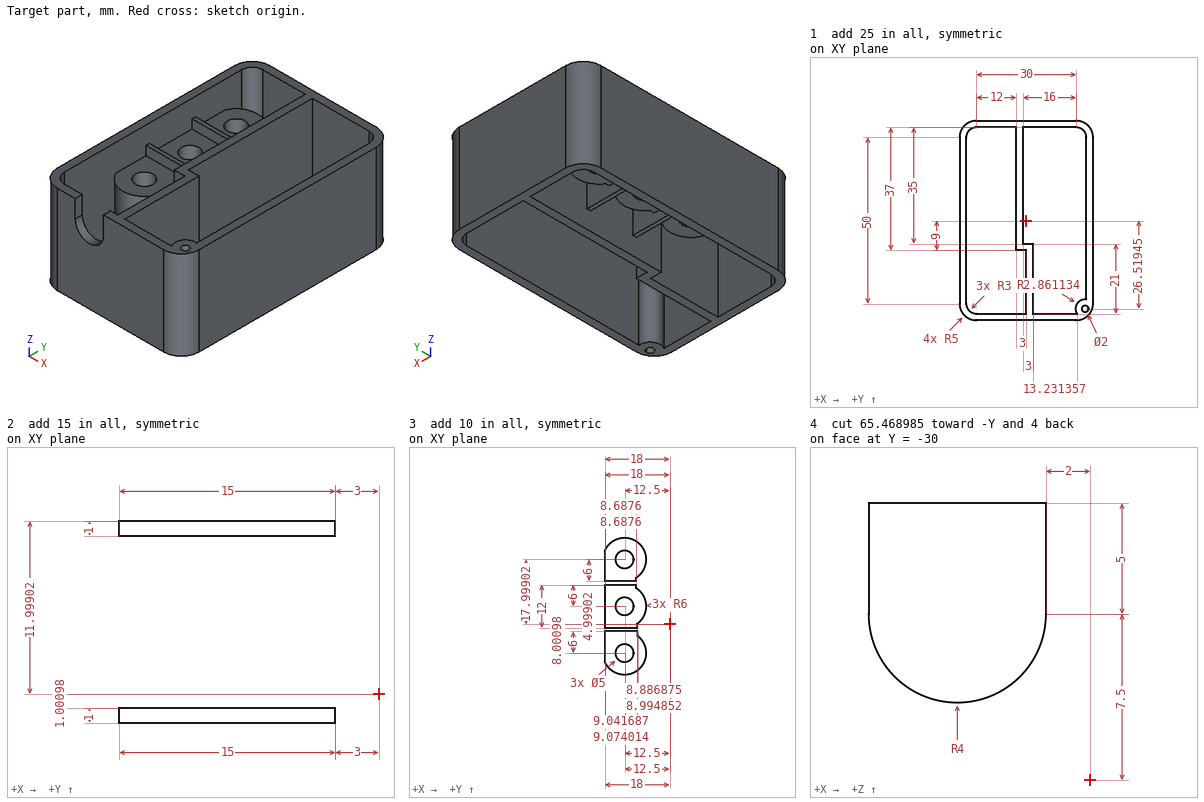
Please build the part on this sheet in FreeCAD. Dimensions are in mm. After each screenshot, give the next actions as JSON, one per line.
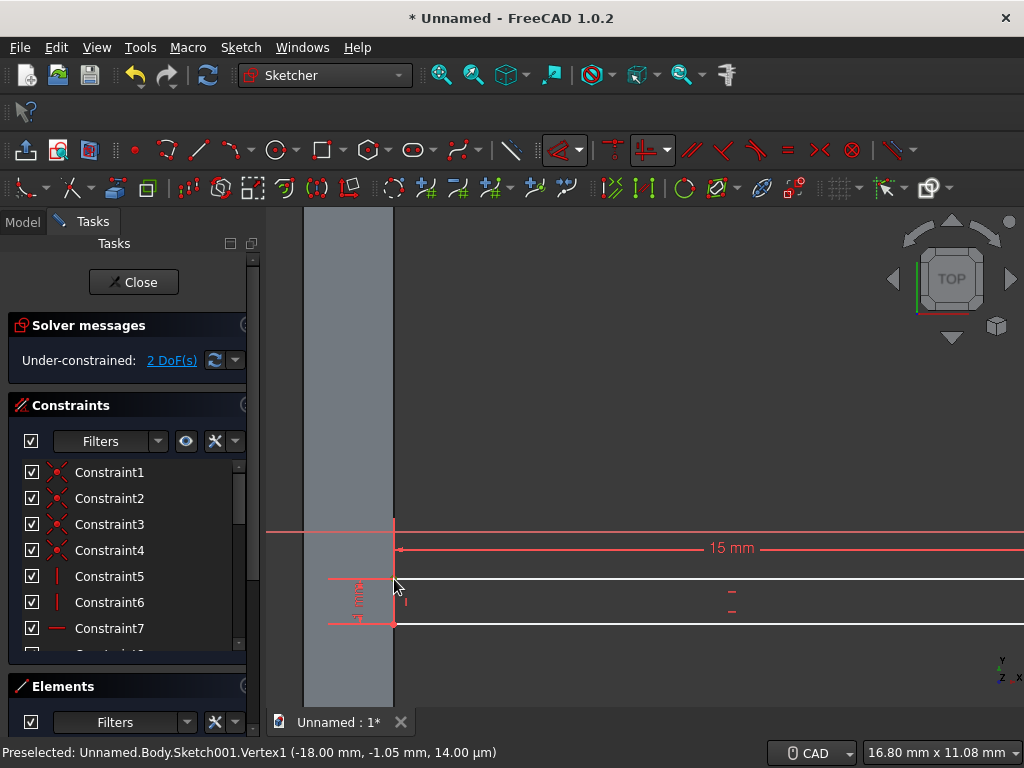
{"action": "key", "text": "i"}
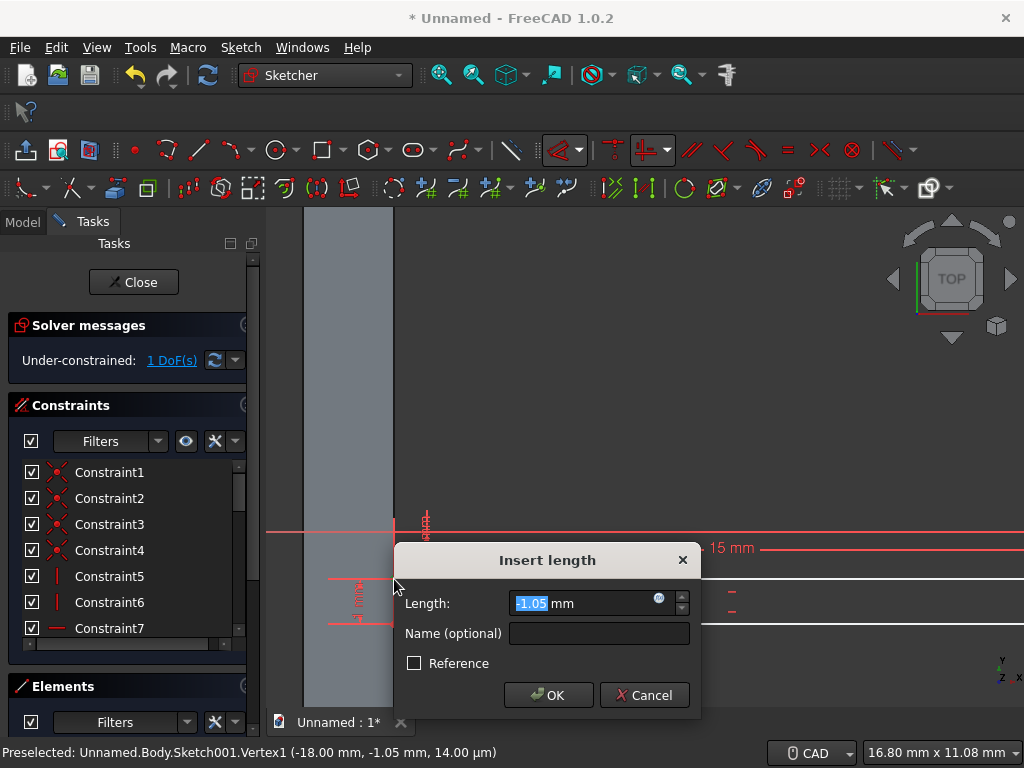
{"action": "type", "text": "-1.00098"}
{"action": "key", "text": "Return"}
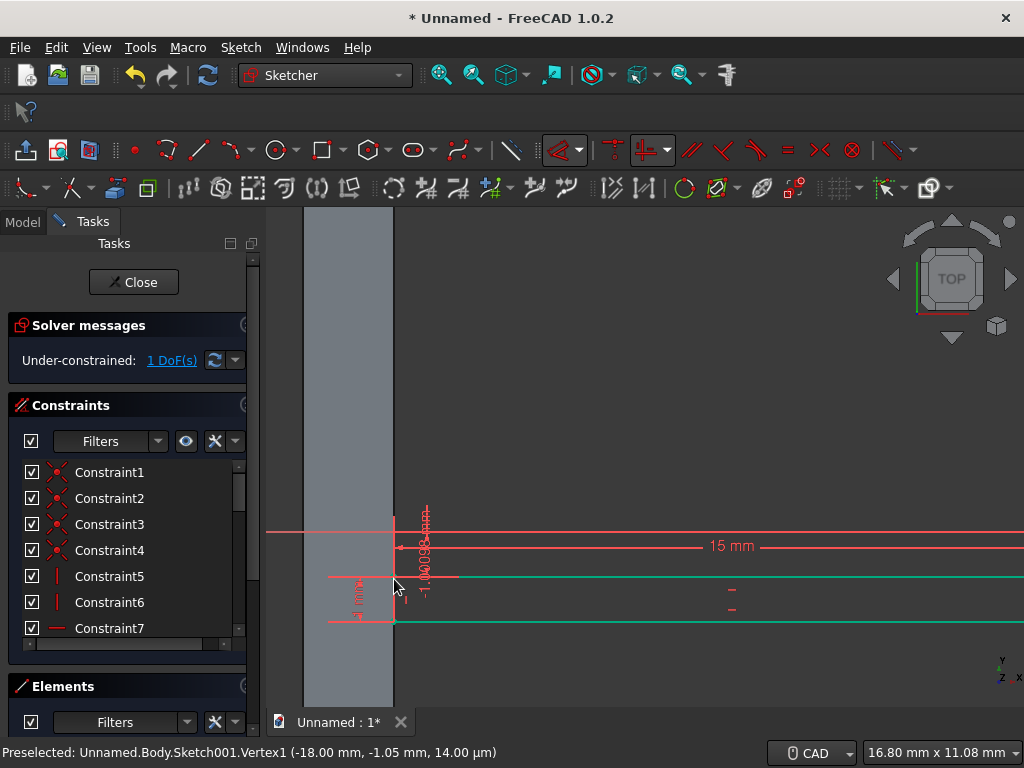
{"action": "scroll", "coordinate": [394, 580], "scroll_direction": "down", "scroll_amount": 4}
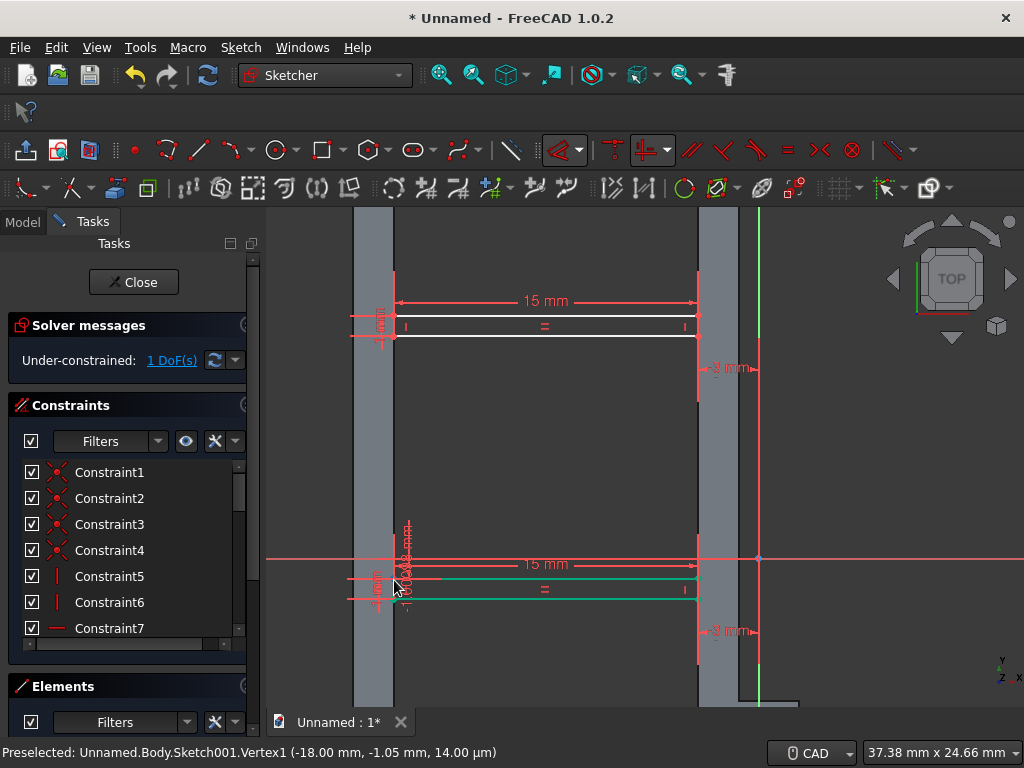
{"action": "left_click", "coordinate": [394, 316]}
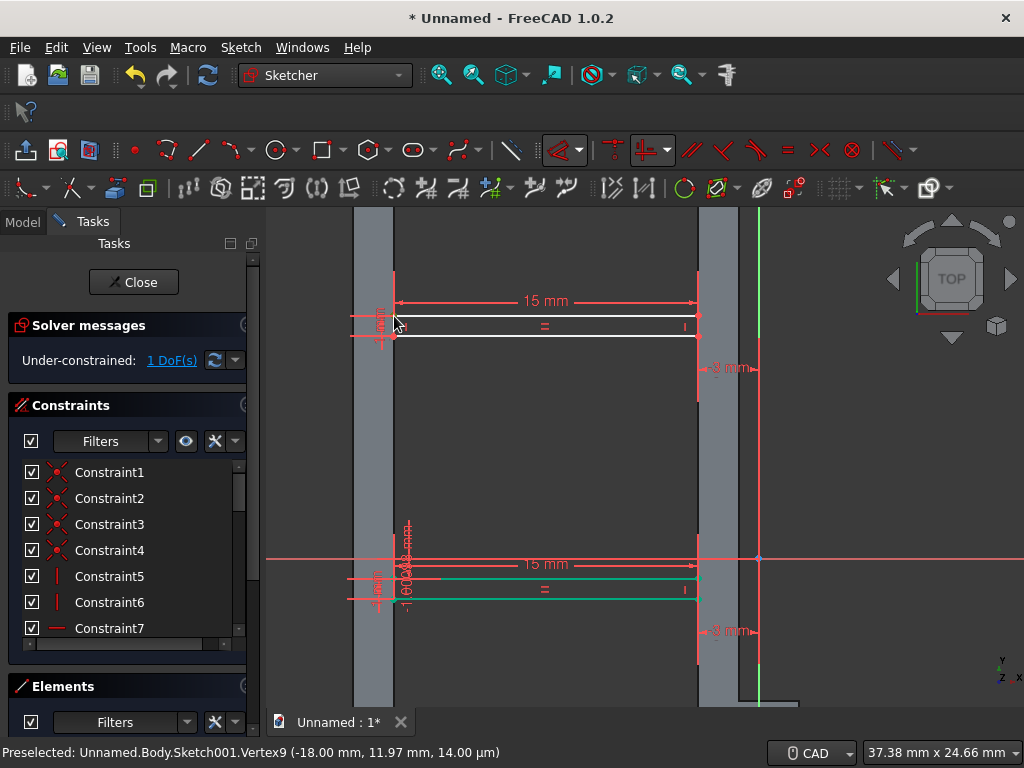
{"action": "left_click", "coordinate": [582, 150]}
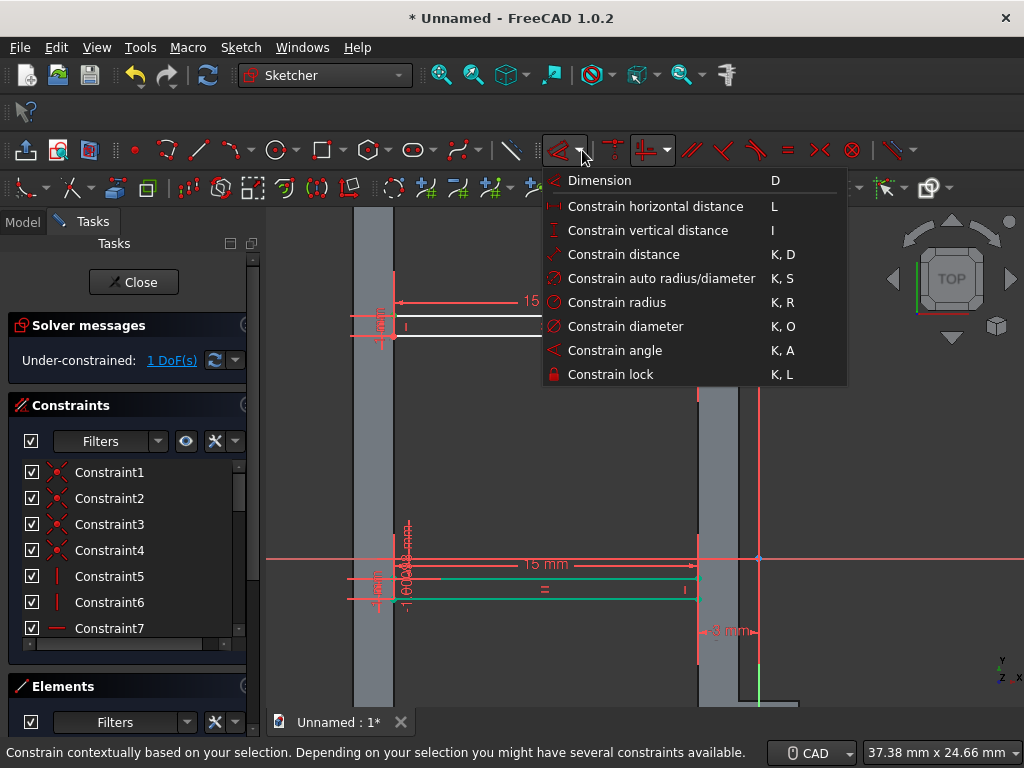
{"action": "left_click", "coordinate": [695, 230]}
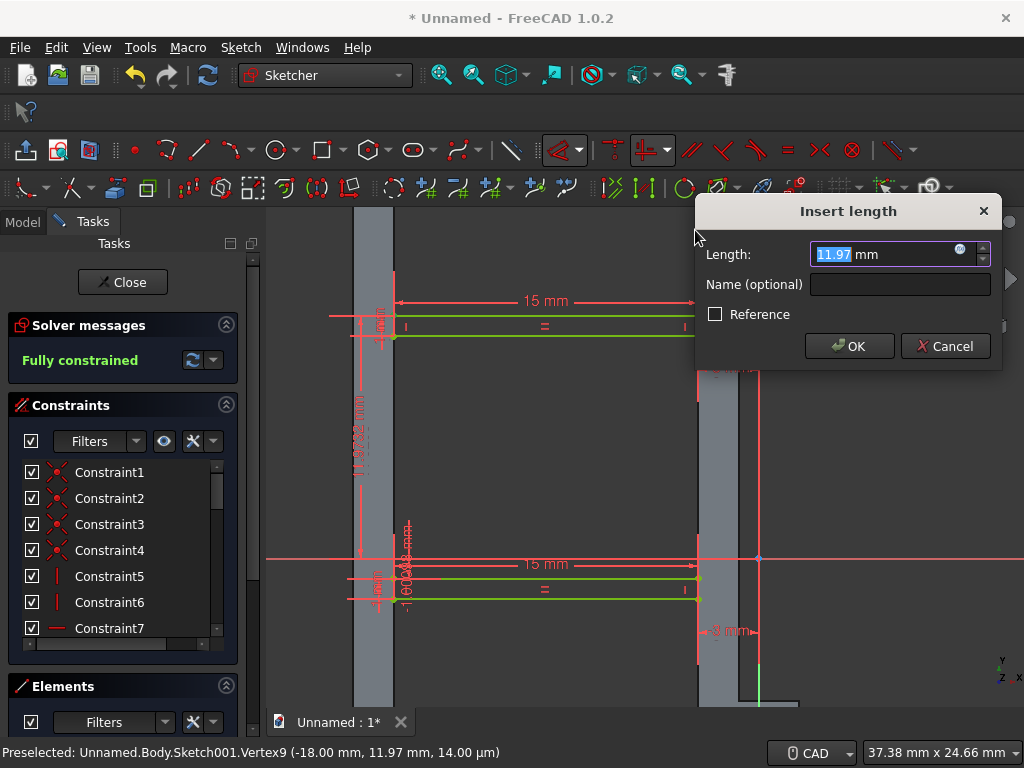
{"action": "type", "text": "11.99902"}
{"action": "key", "text": "Return"}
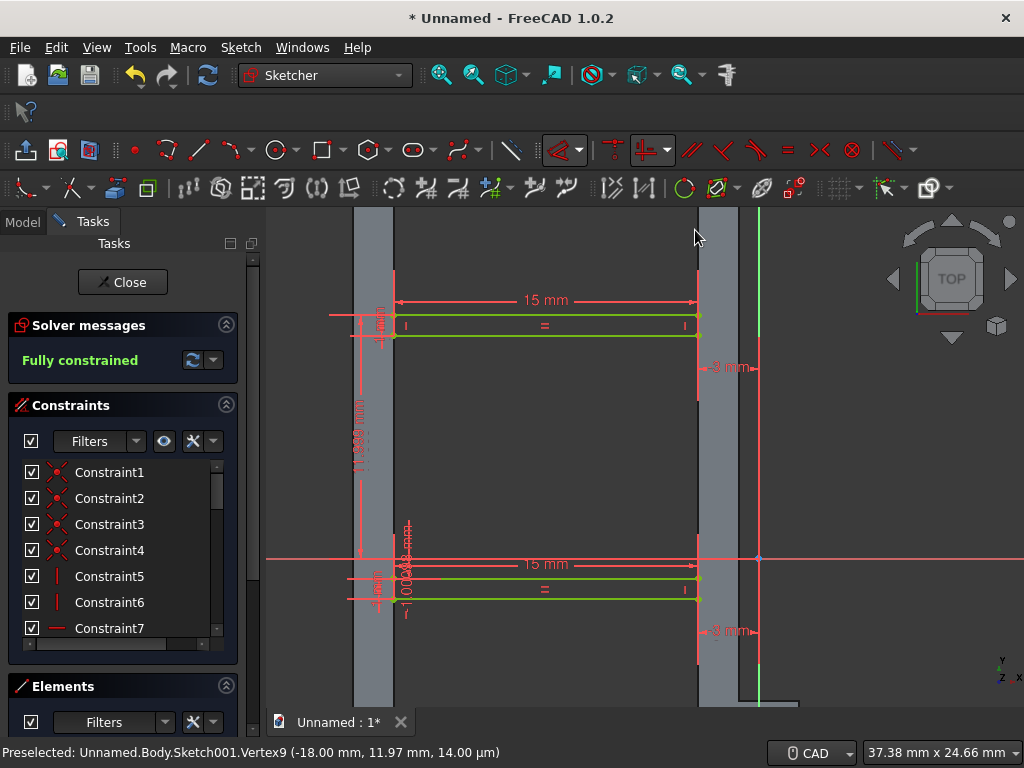
{"action": "left_click", "coordinate": [123, 282]}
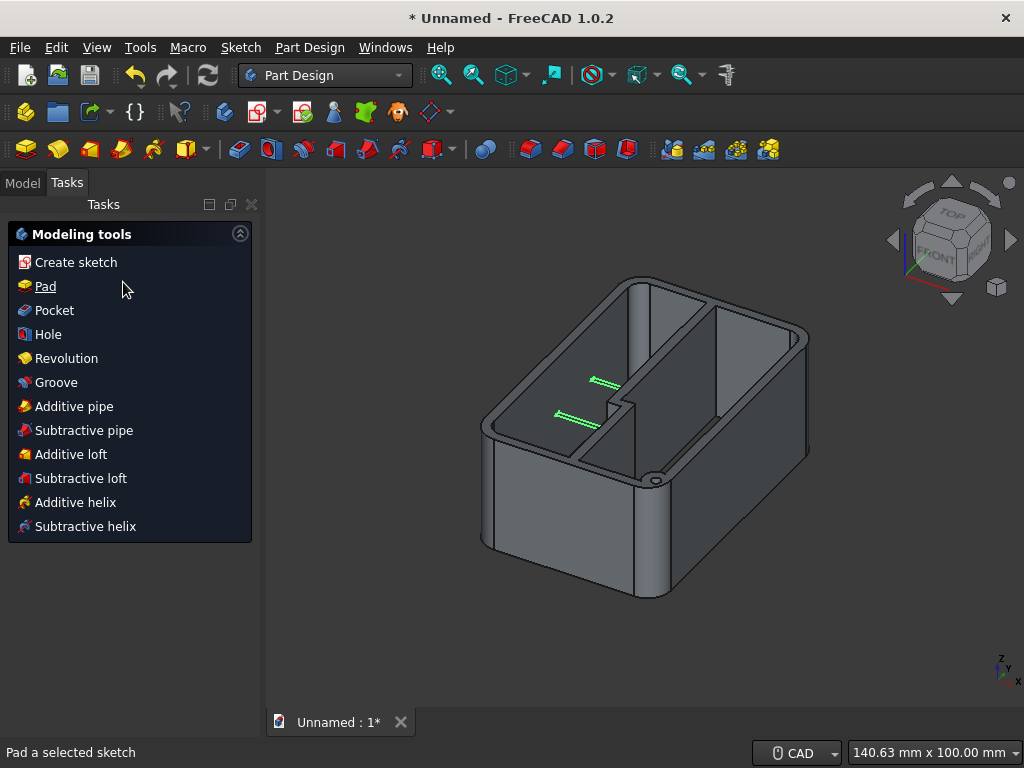
{"action": "left_click", "coordinate": [26, 150]}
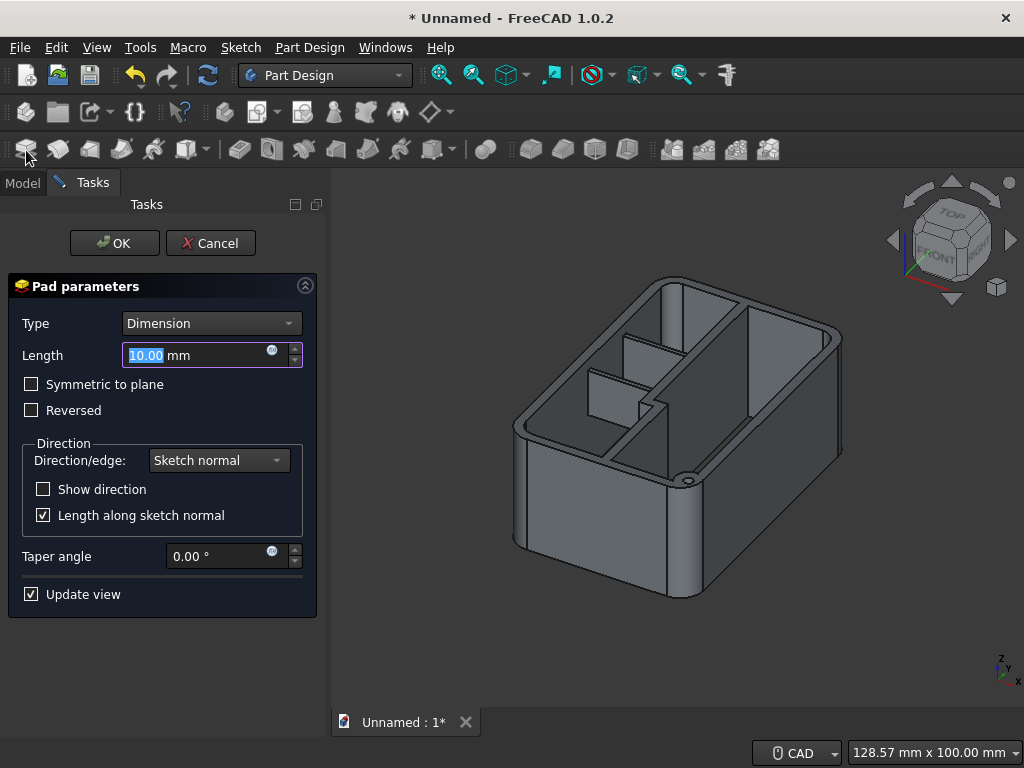
{"action": "type", "text": "15"}
{"action": "key", "text": "Tab"}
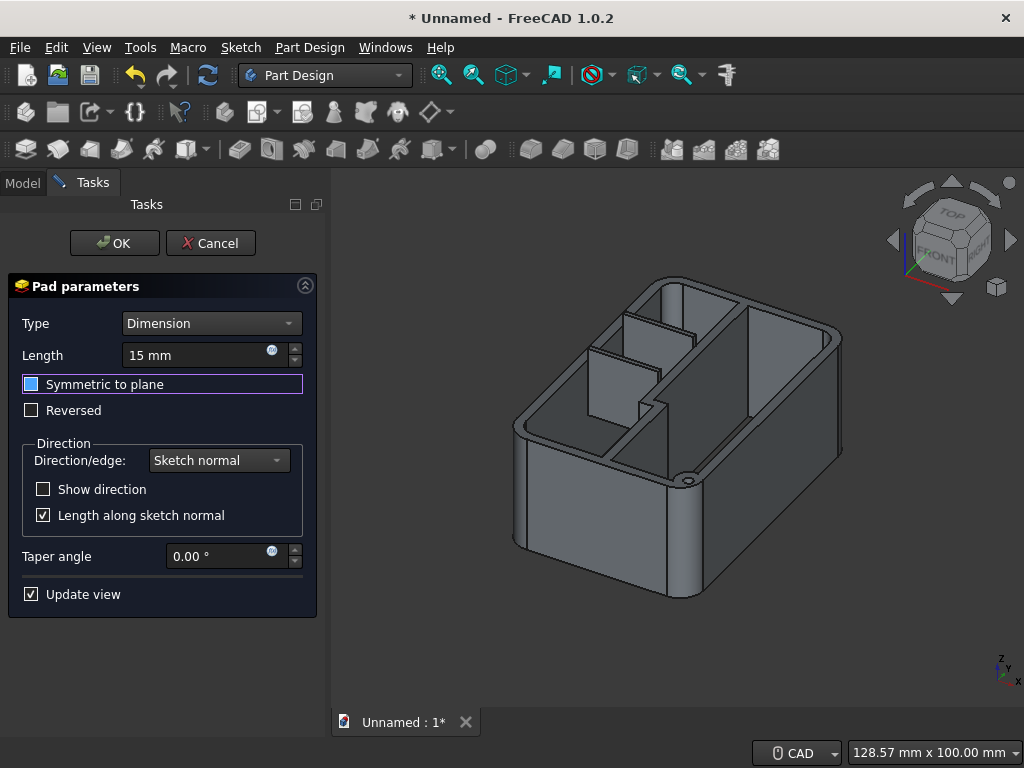
{"action": "left_click", "coordinate": [30, 384]}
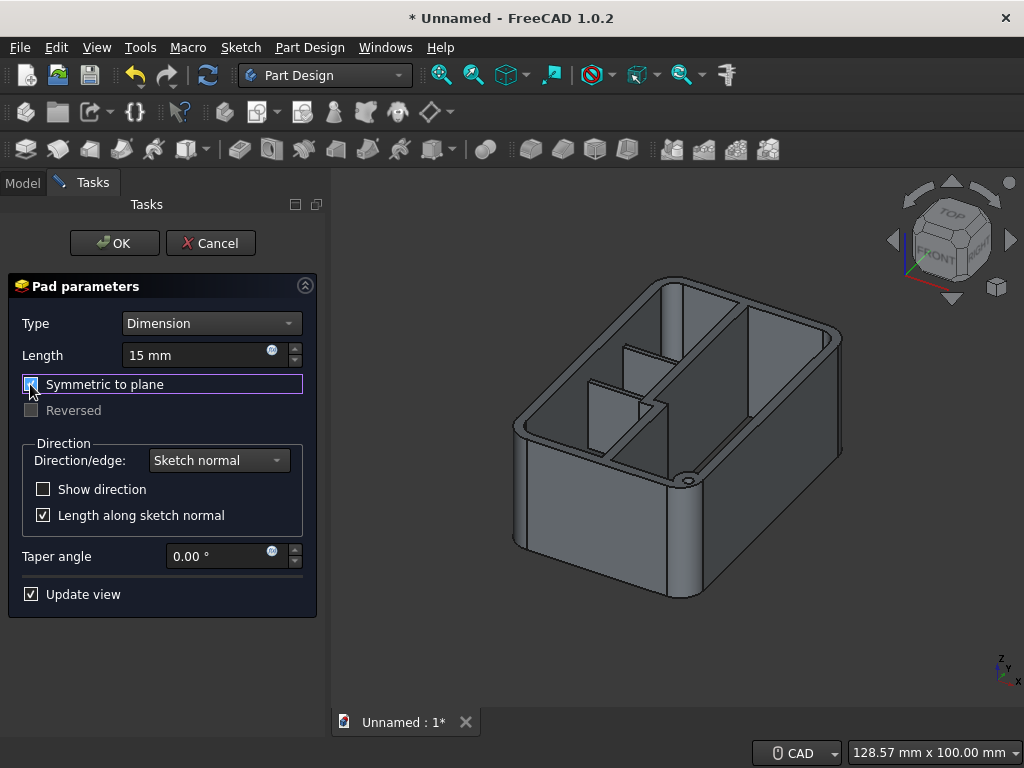
{"action": "left_click", "coordinate": [115, 243]}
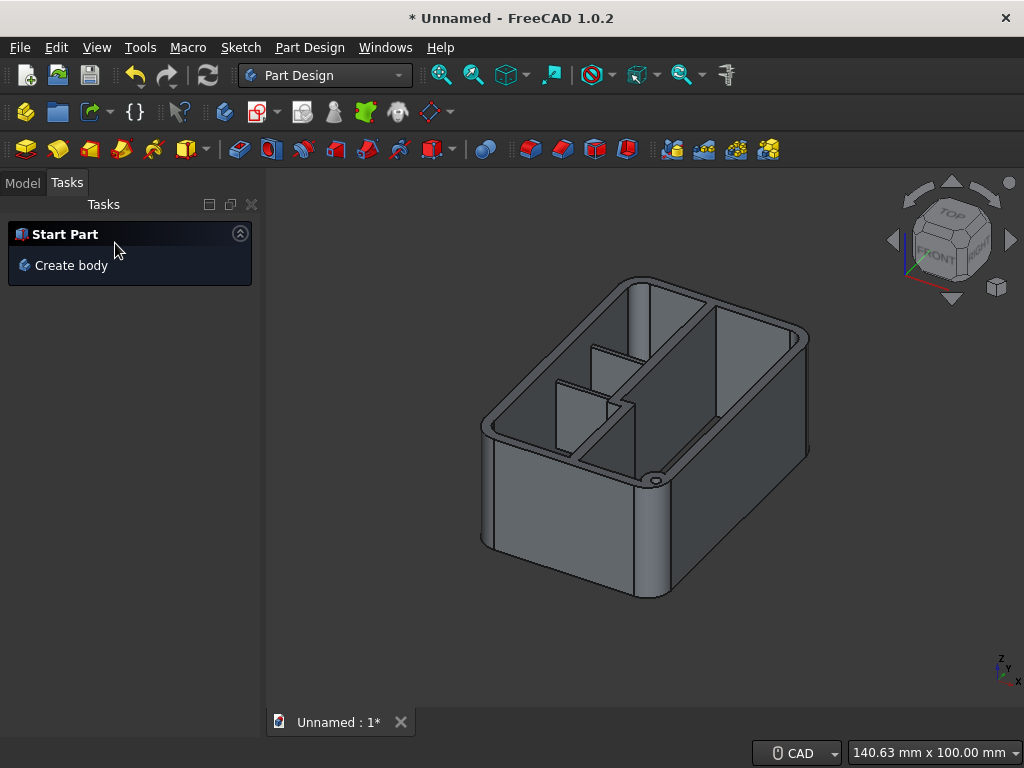
{"action": "left_click", "coordinate": [258, 112]}